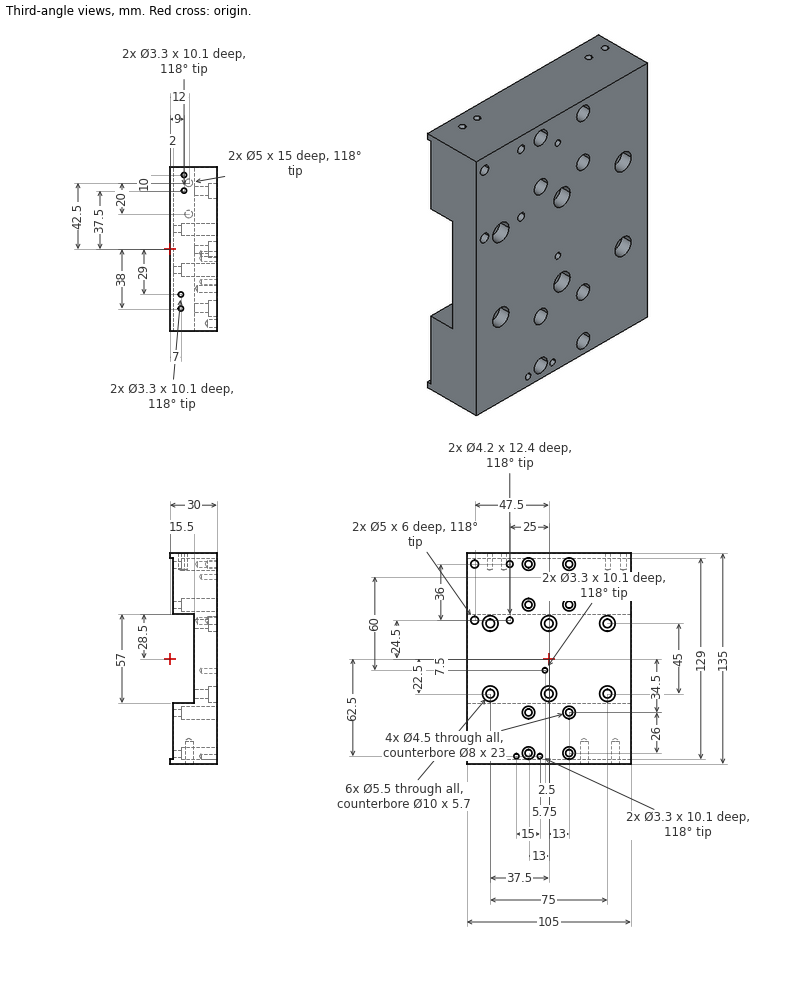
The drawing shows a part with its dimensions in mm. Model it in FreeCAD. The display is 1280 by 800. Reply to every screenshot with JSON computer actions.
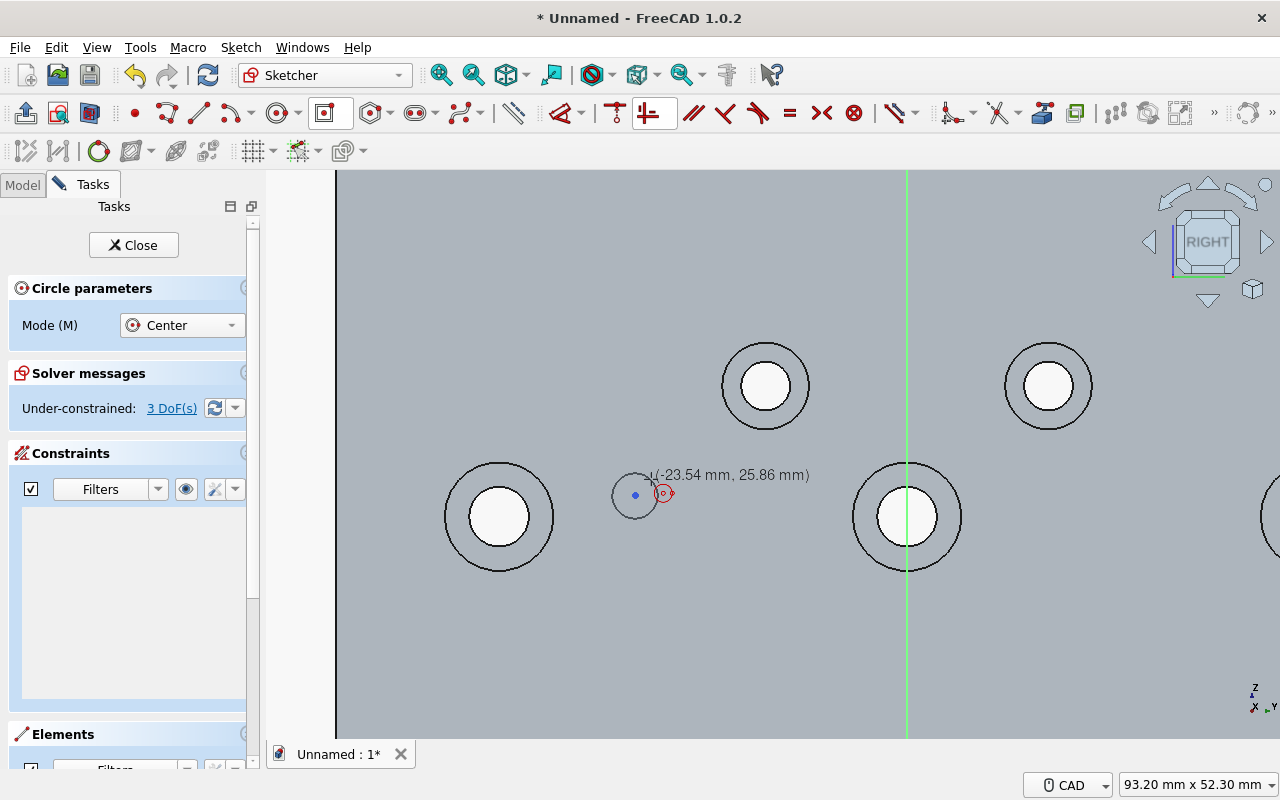
{"action": "scroll", "coordinate": [637, 495], "scroll_direction": "down", "scroll_amount": 3}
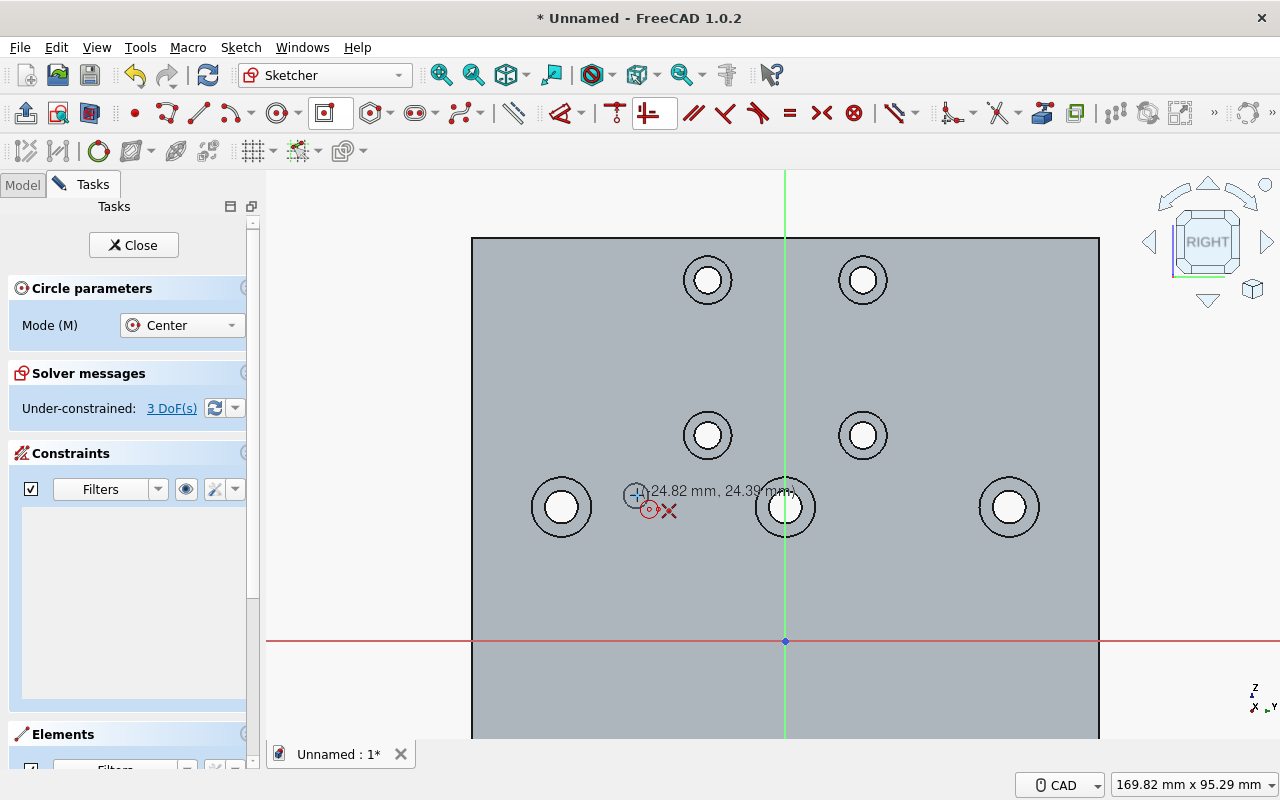
{"action": "scroll", "coordinate": [636, 280], "scroll_direction": "up", "scroll_amount": 3}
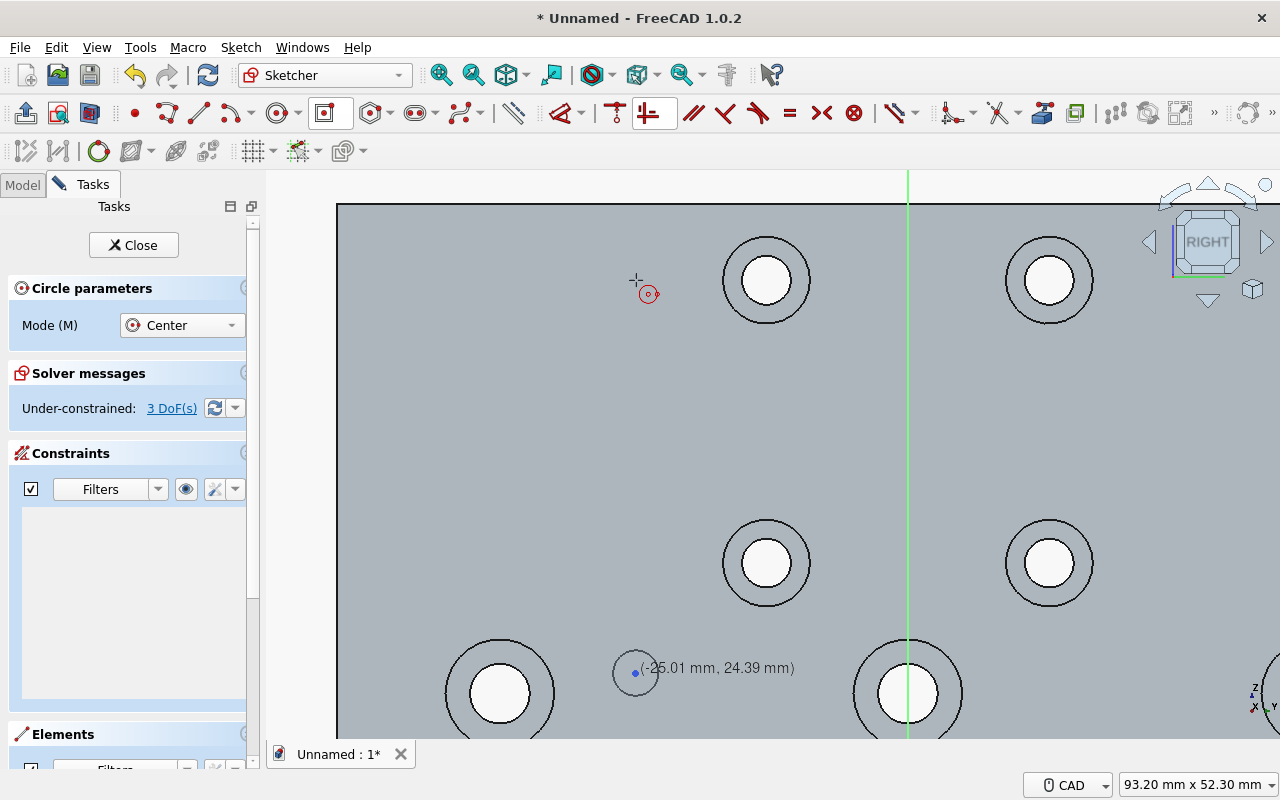
{"action": "left_click", "coordinate": [636, 280]}
{"action": "left_click", "coordinate": [652, 264]}
{"action": "key", "text": "Escape"}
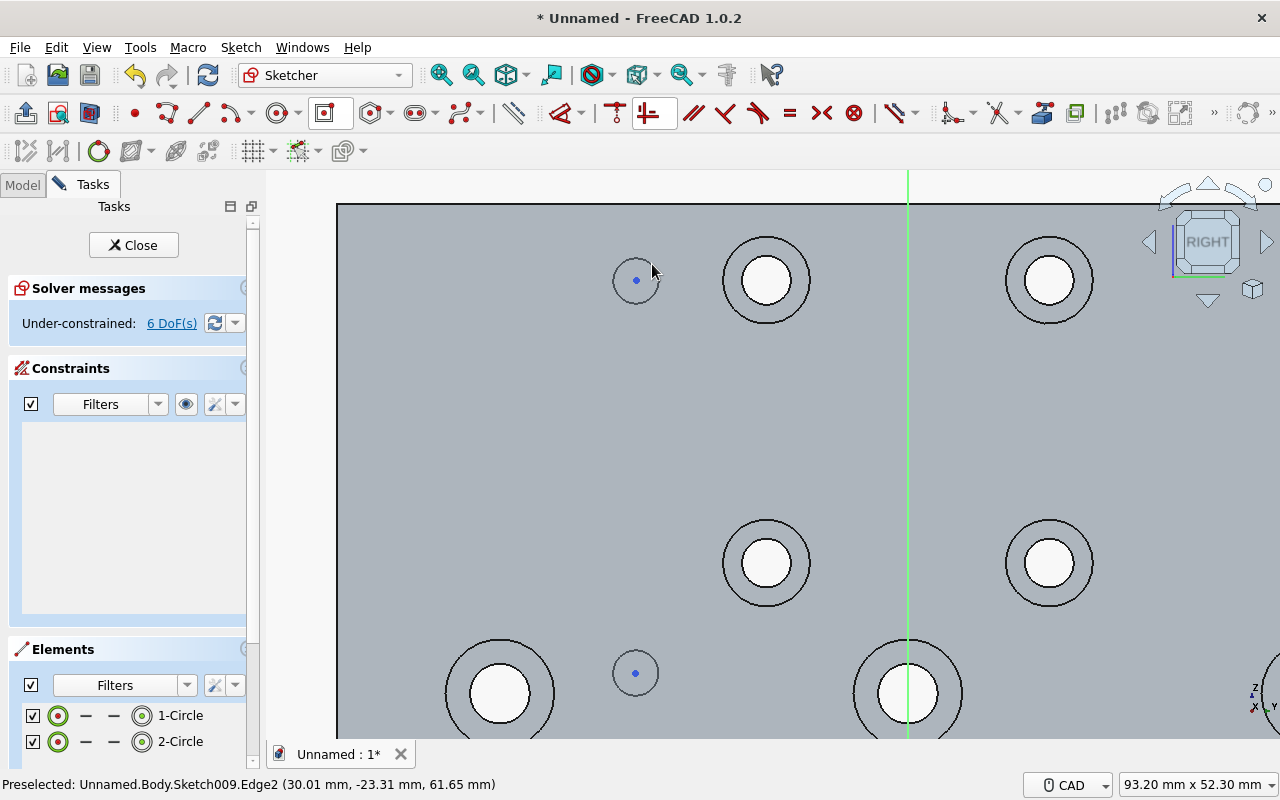
{"action": "left_click", "coordinate": [652, 657]}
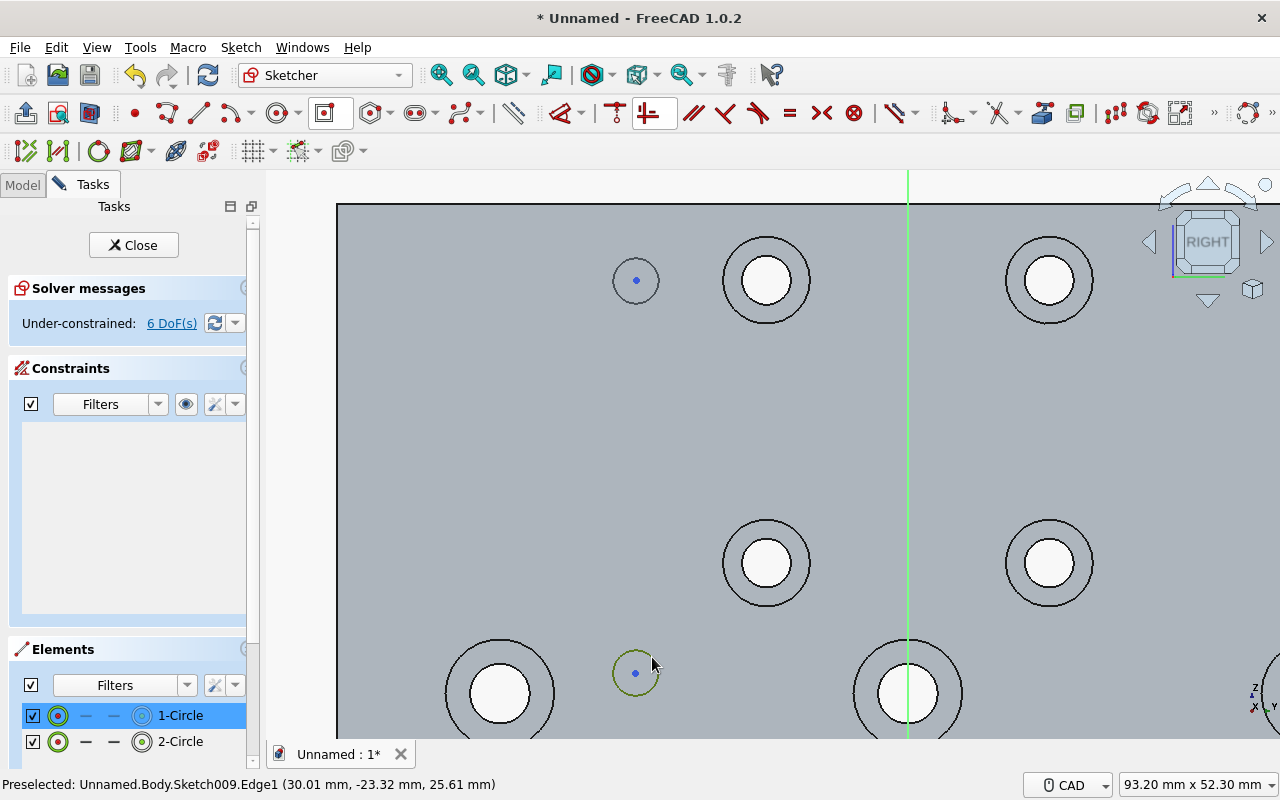
{"action": "left_click", "coordinate": [652, 265]}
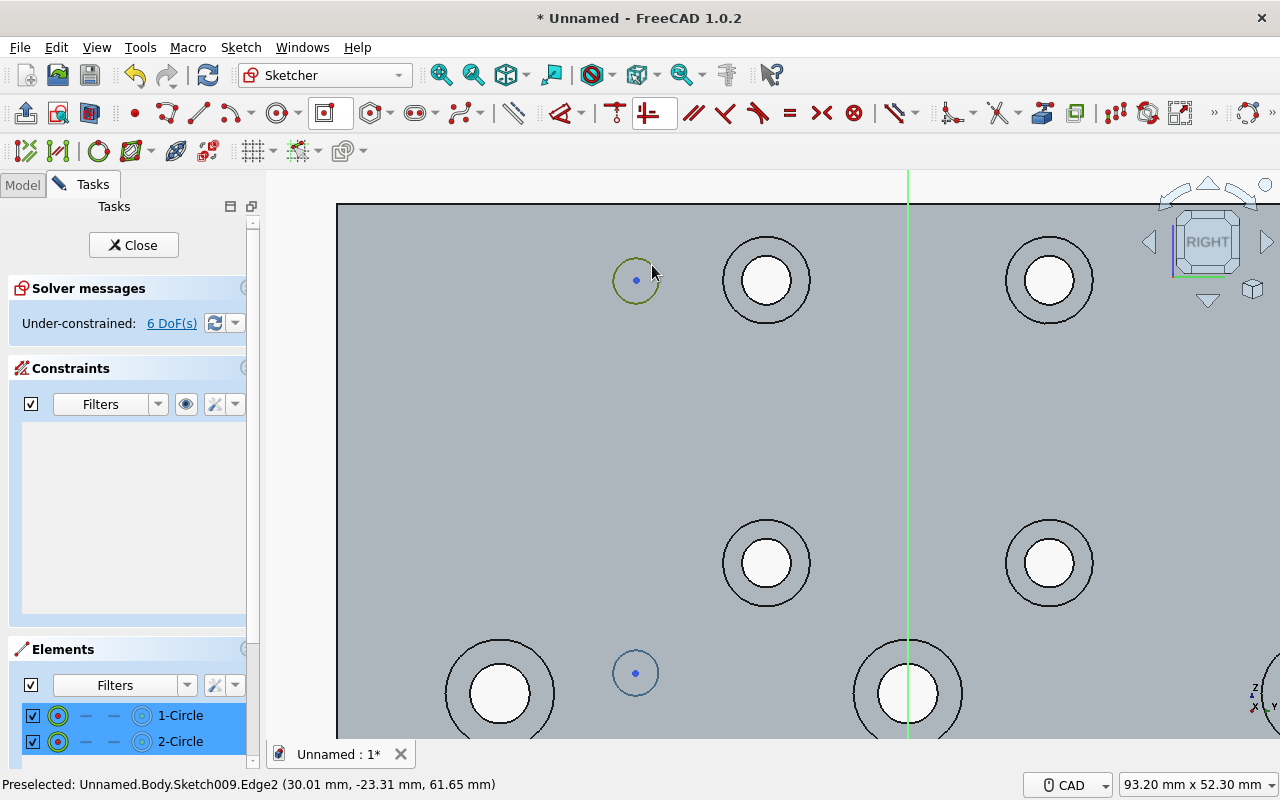
{"action": "left_click", "coordinate": [790, 114]}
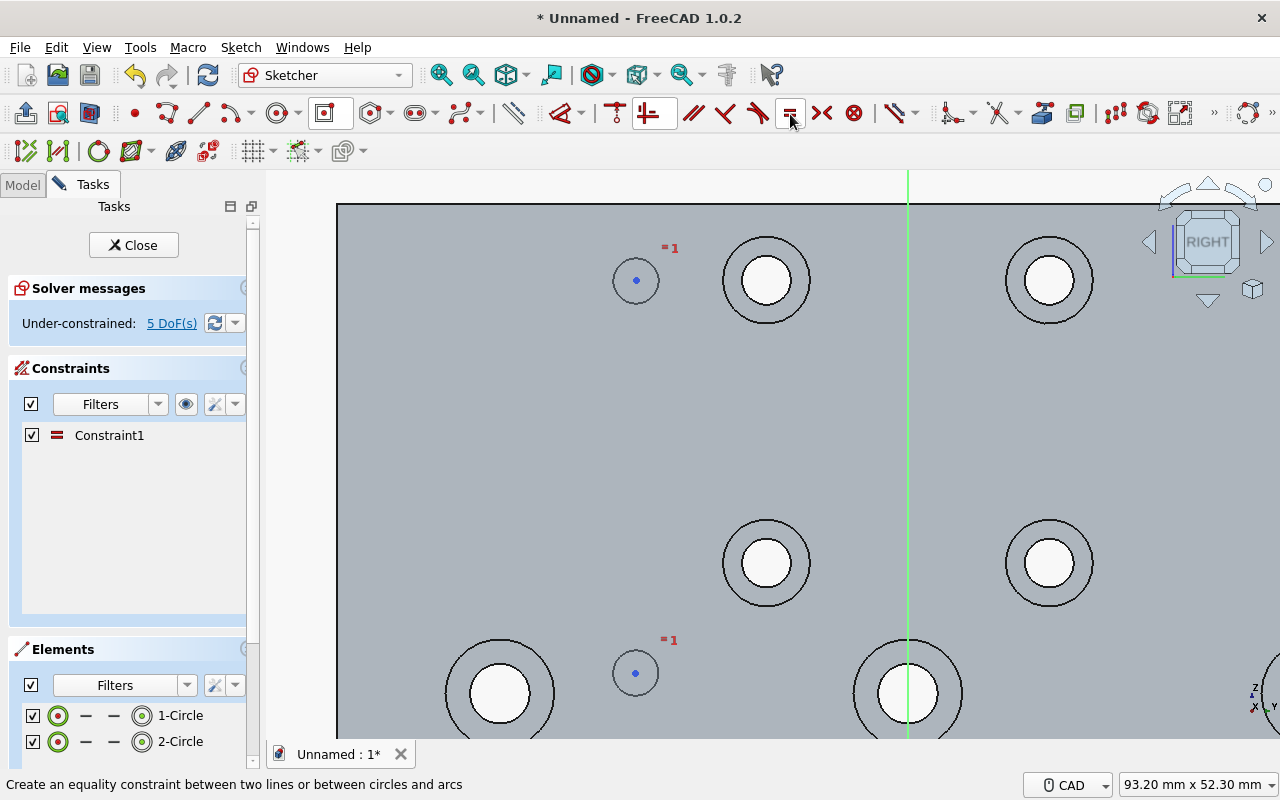
{"action": "left_click", "coordinate": [636, 673]}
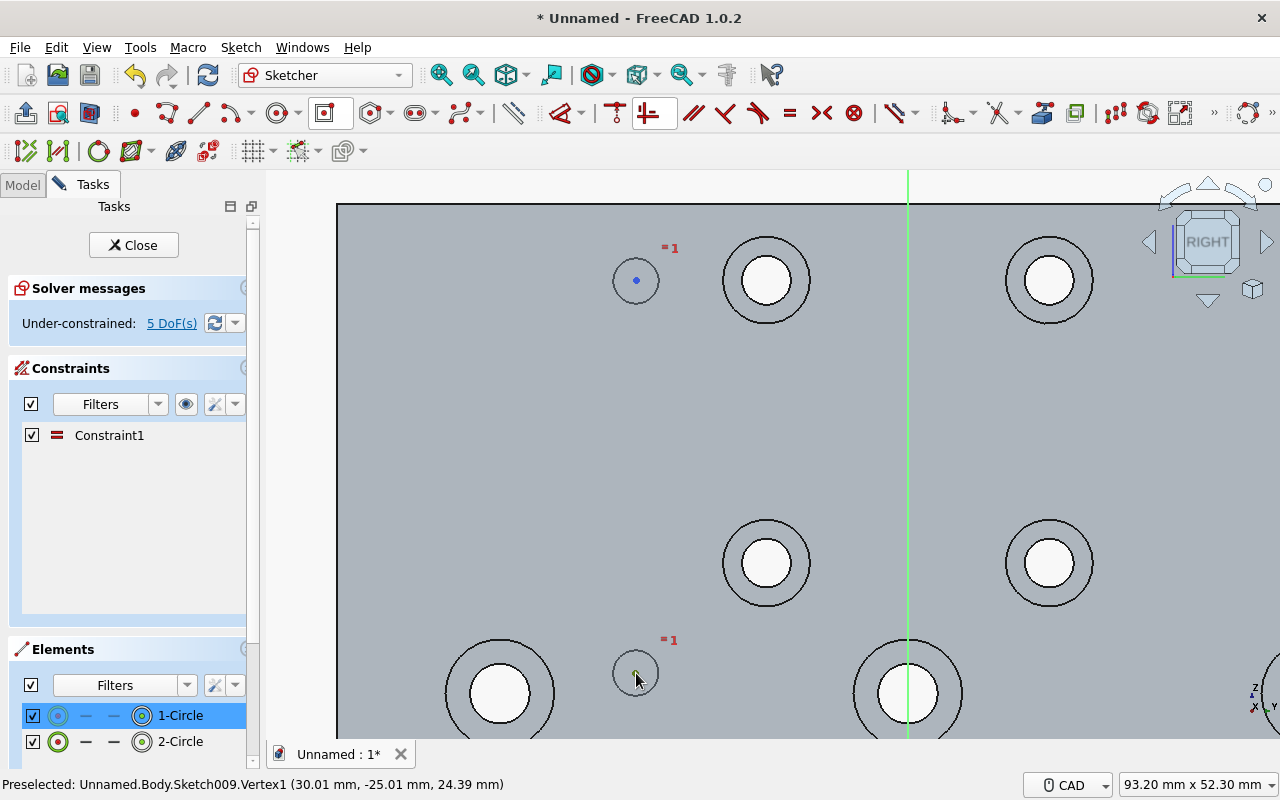
{"action": "left_click", "coordinate": [636, 281]}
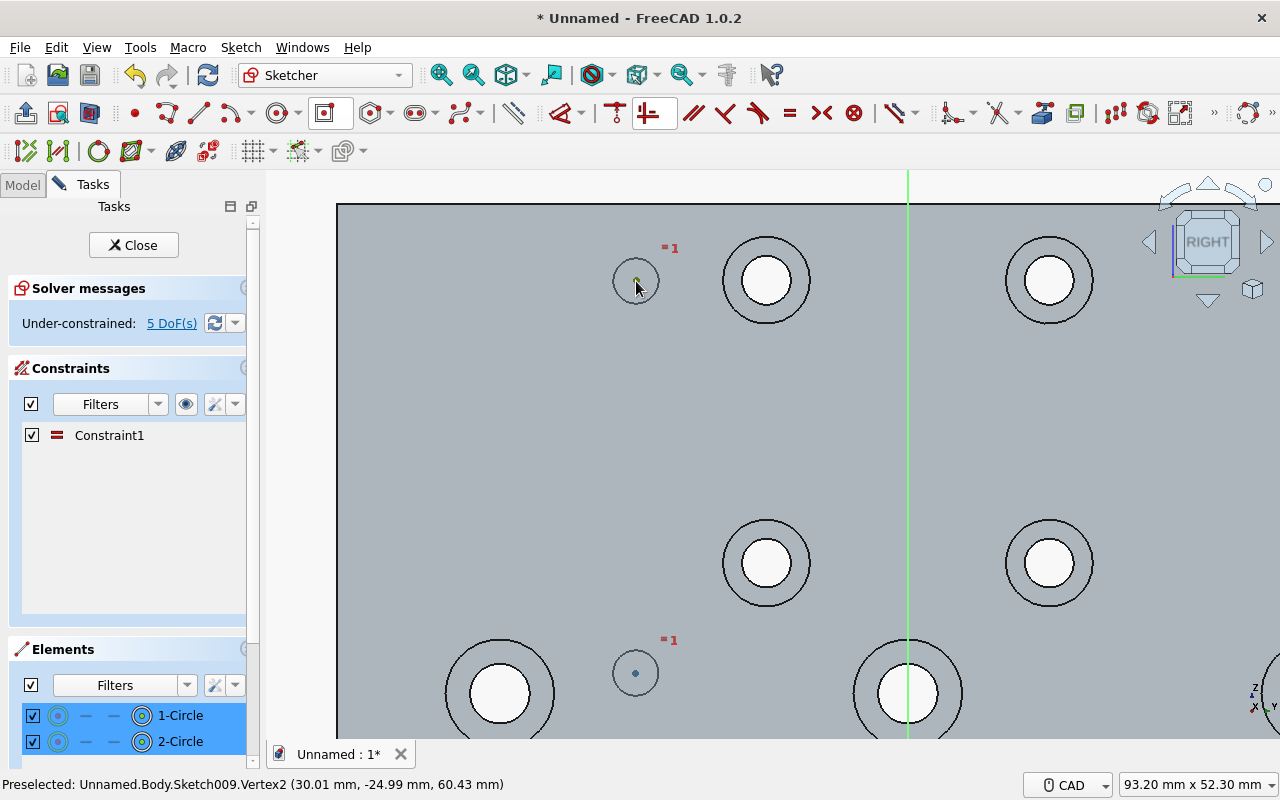
{"action": "key", "text": "v"}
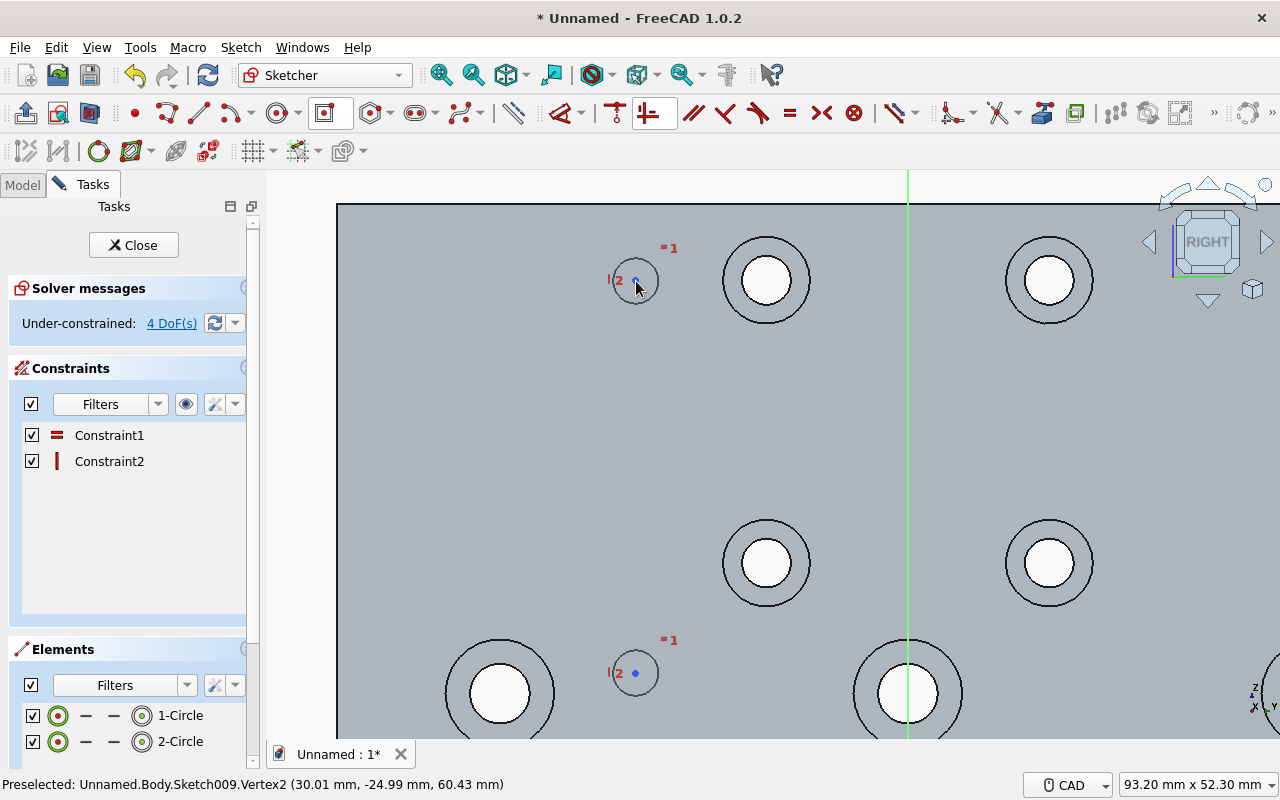
{"action": "left_click", "coordinate": [560, 114]}